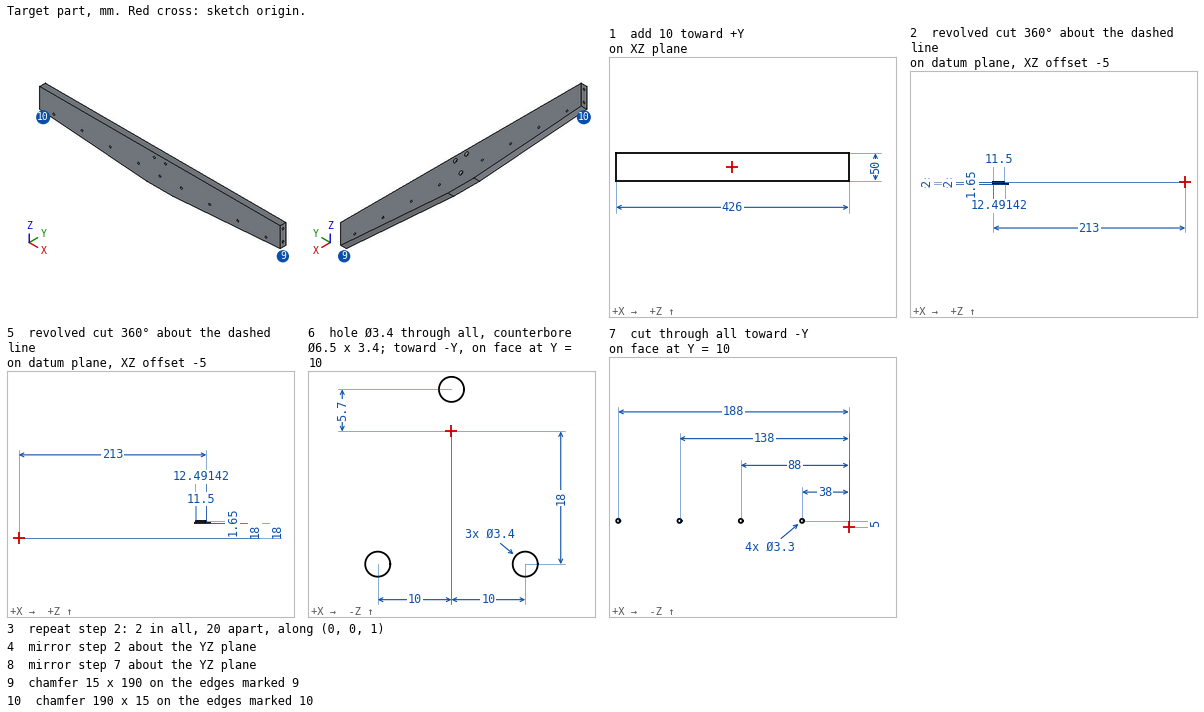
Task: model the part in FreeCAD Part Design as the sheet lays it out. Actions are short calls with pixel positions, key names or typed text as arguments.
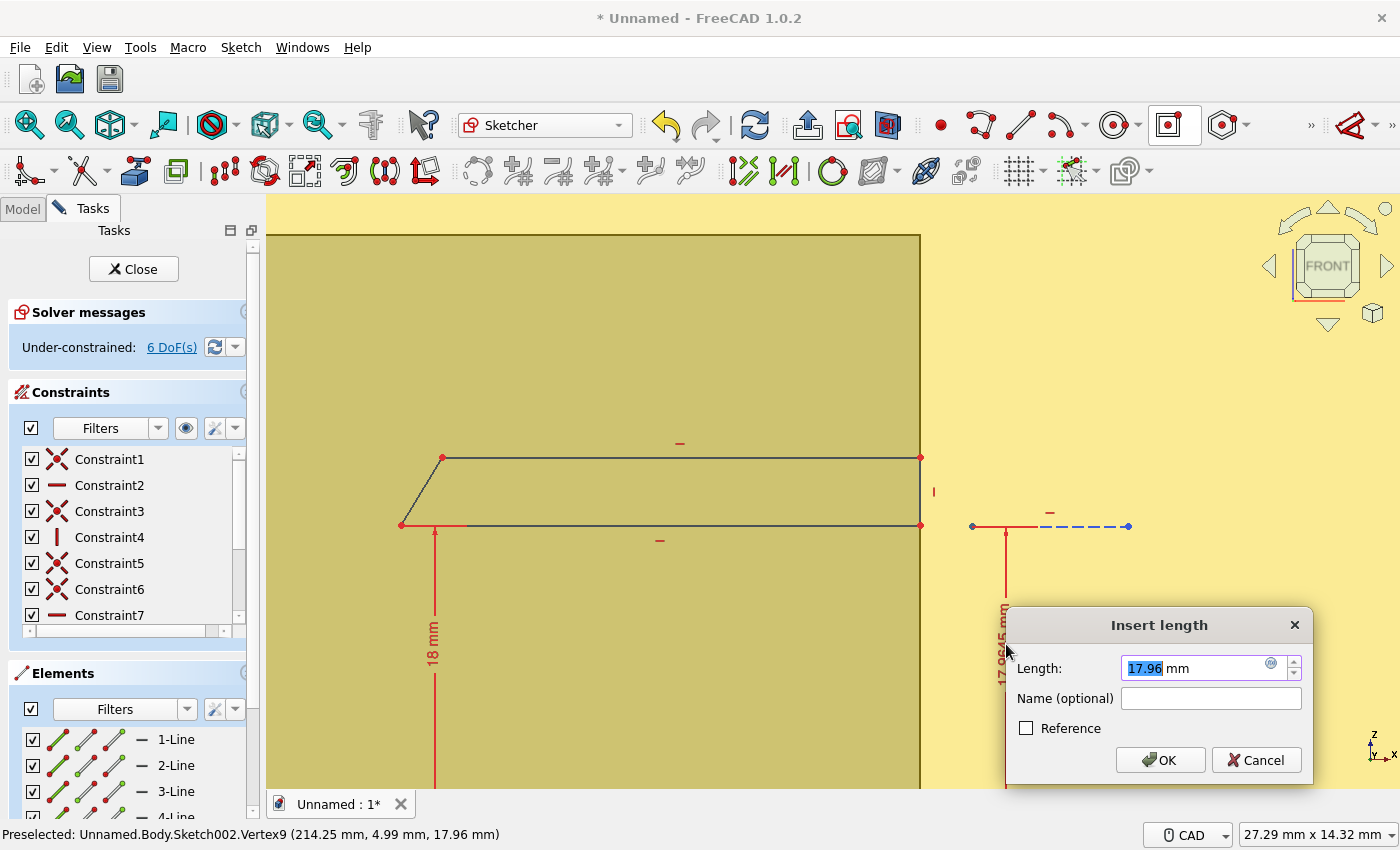
text(18)
key(Return)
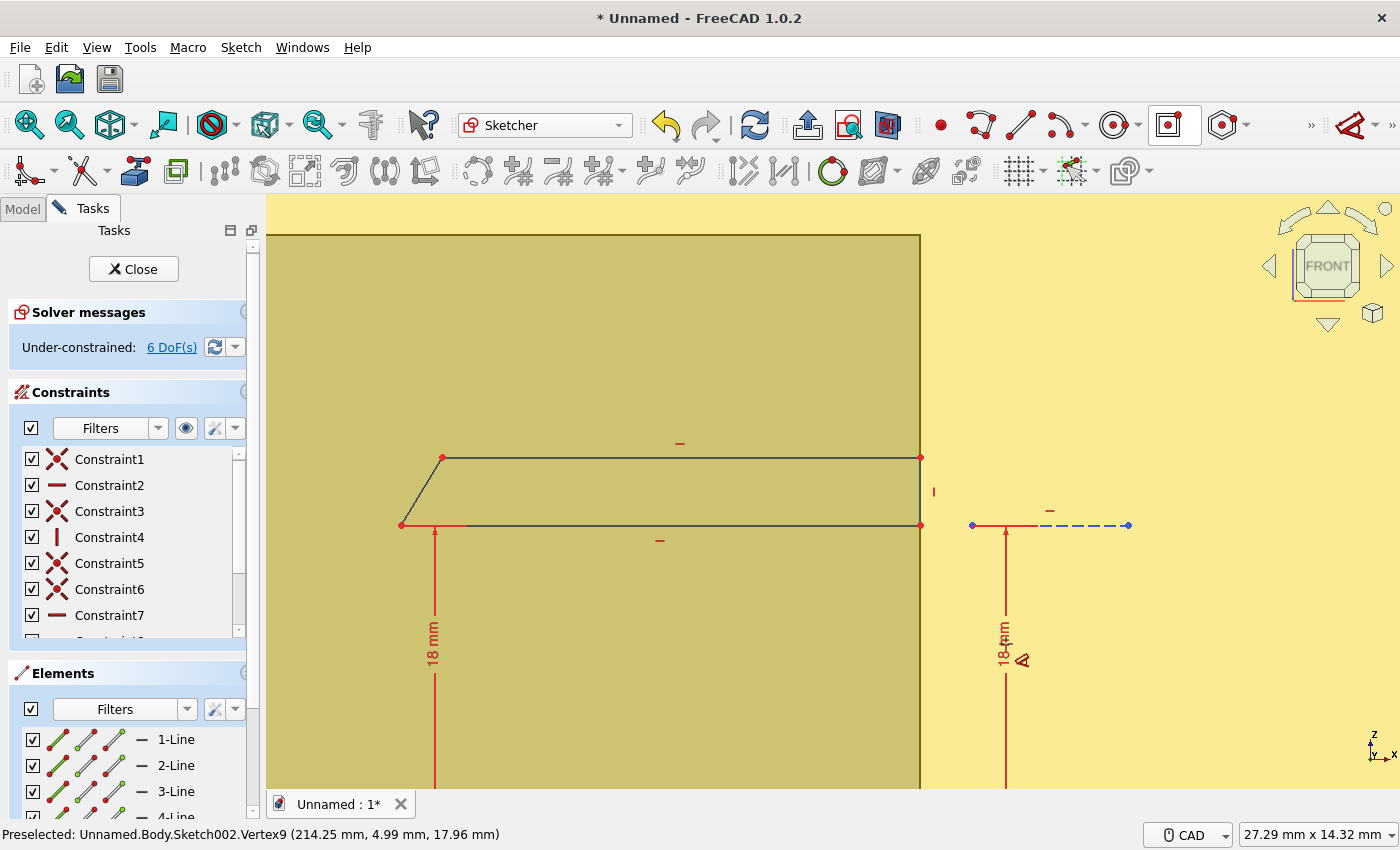
click(585, 458)
click(681, 424)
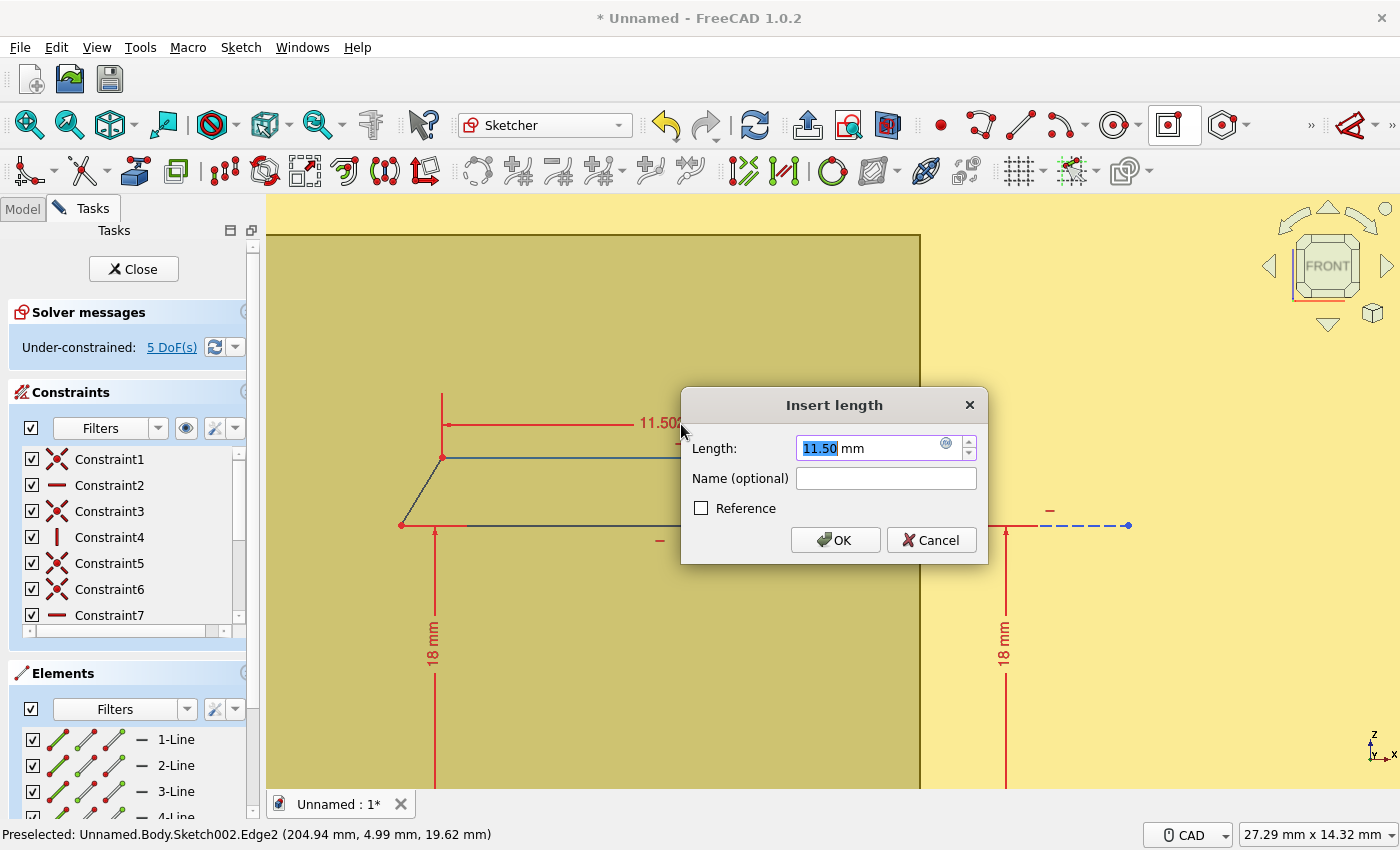
text(11.5)
key(Return)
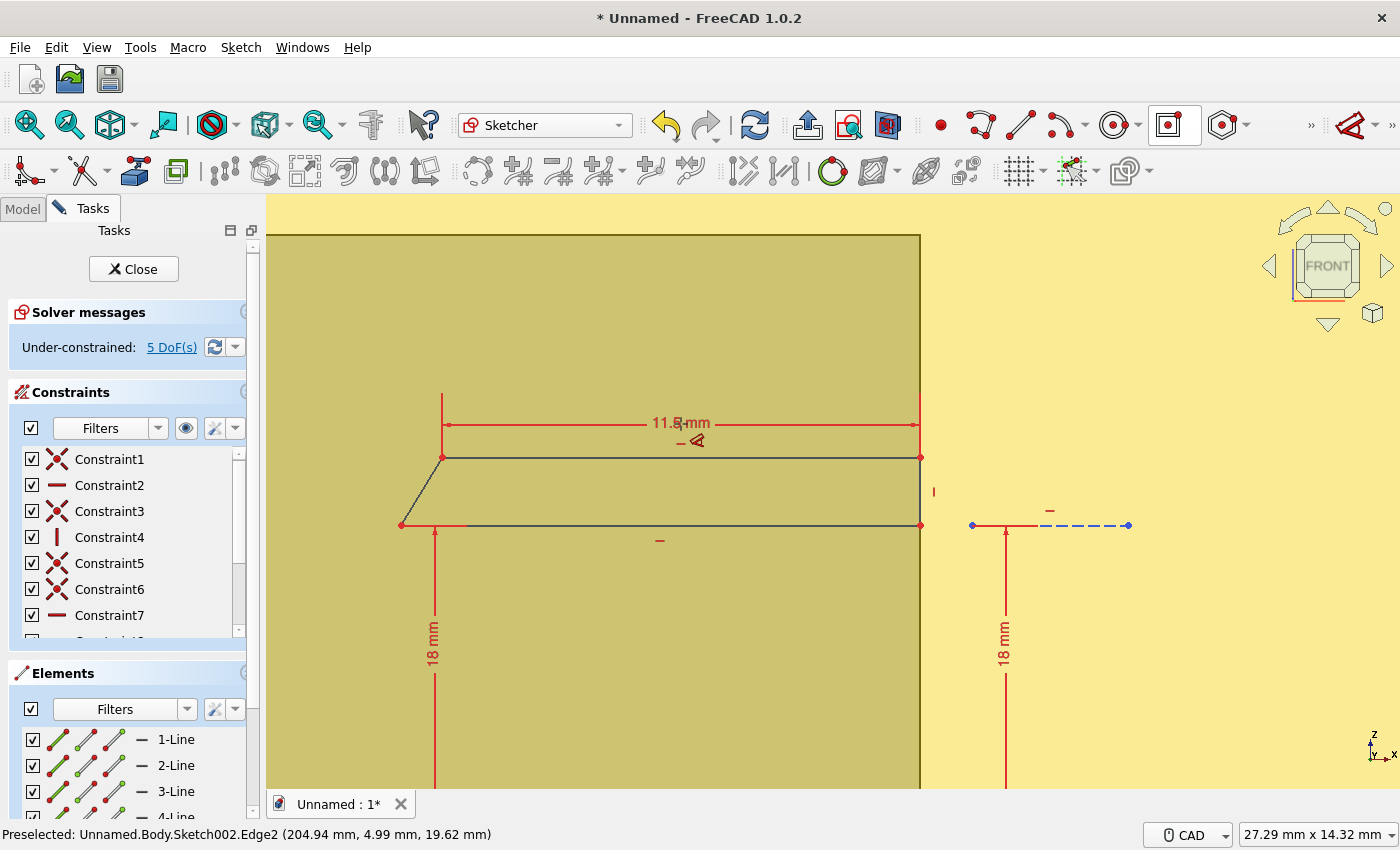
click(920, 478)
click(954, 492)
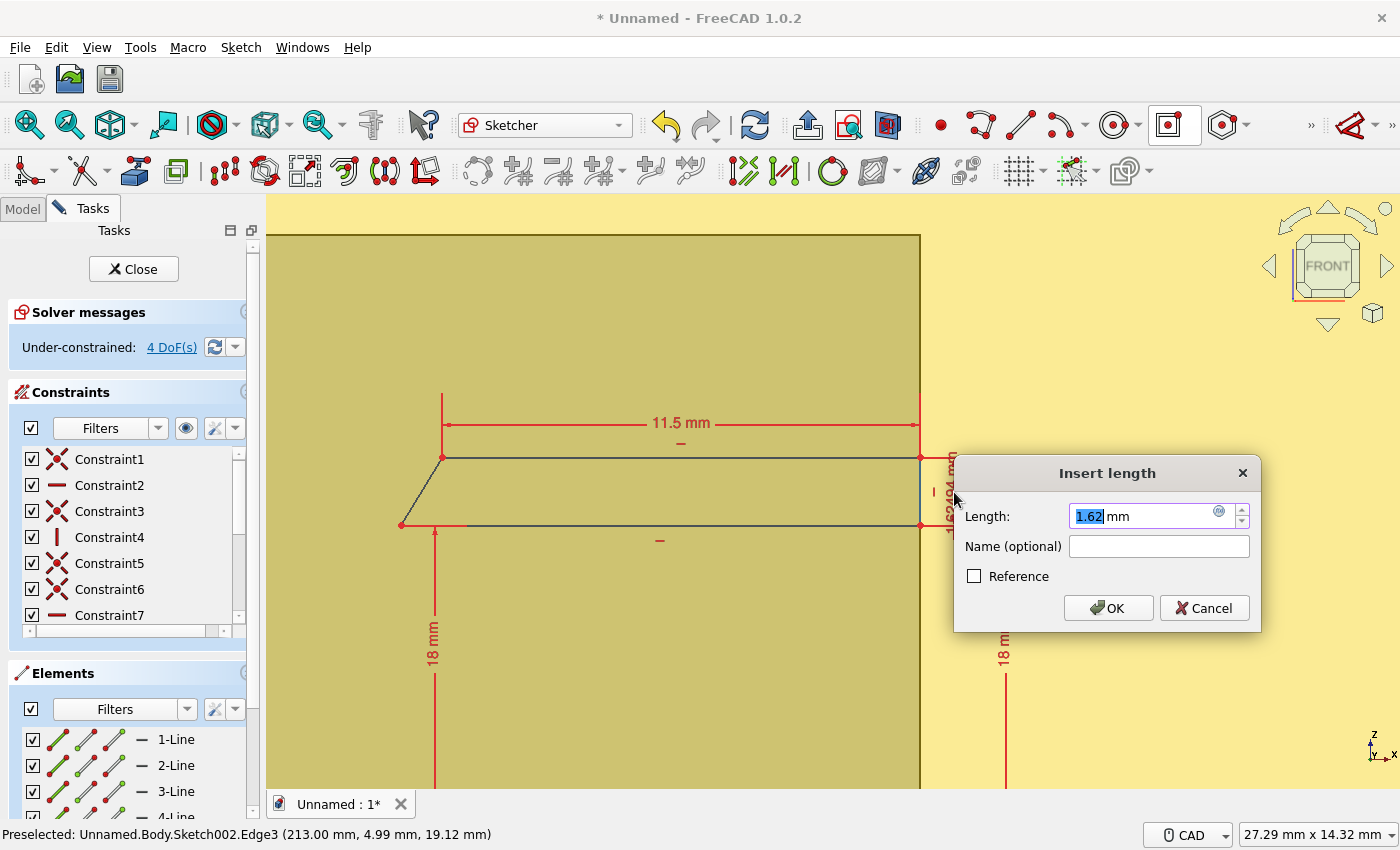
text(1.65)
key(Return)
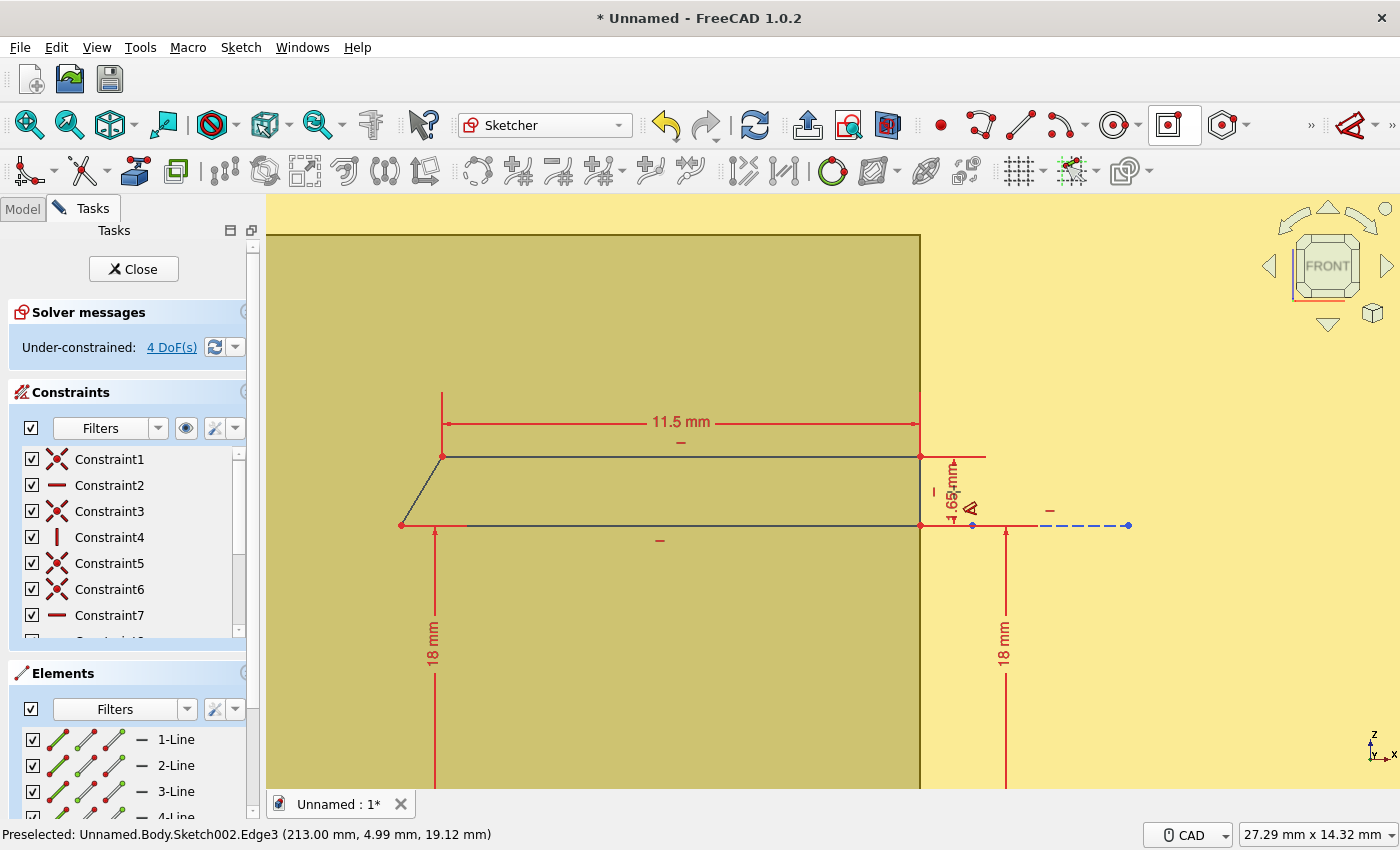
click(920, 457)
click(607, 423)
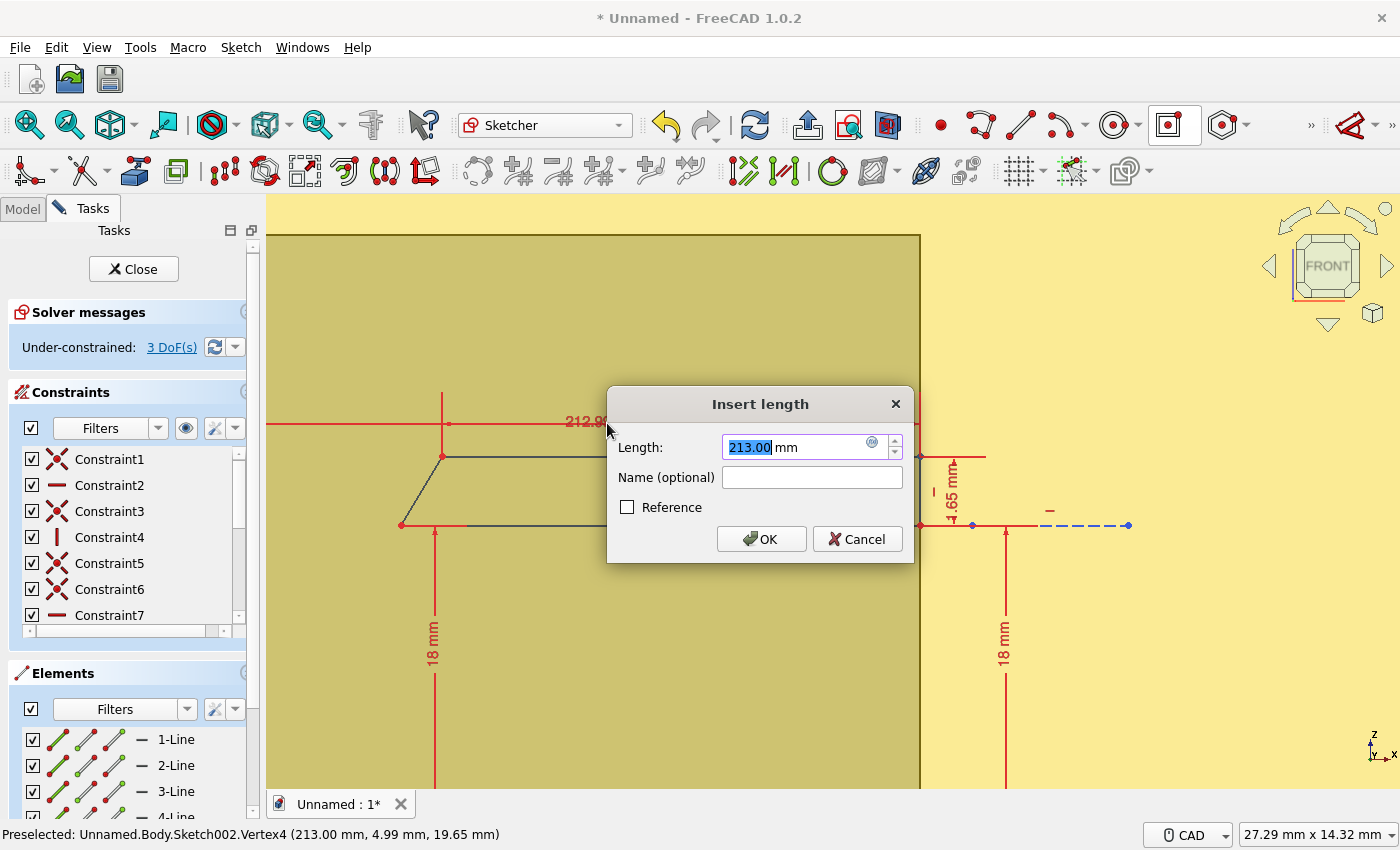
text(213)
key(Return)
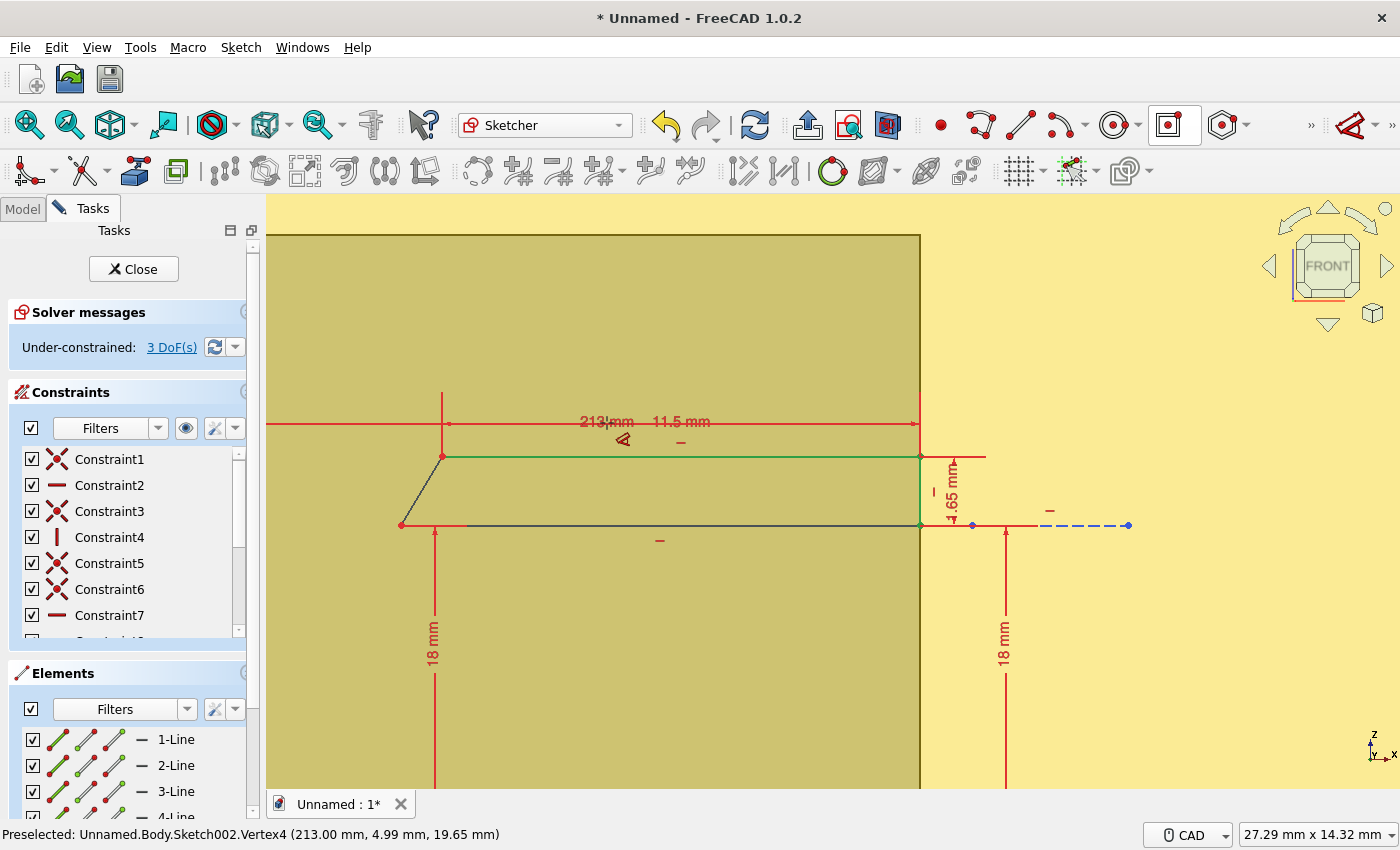
click(764, 526)
click(661, 560)